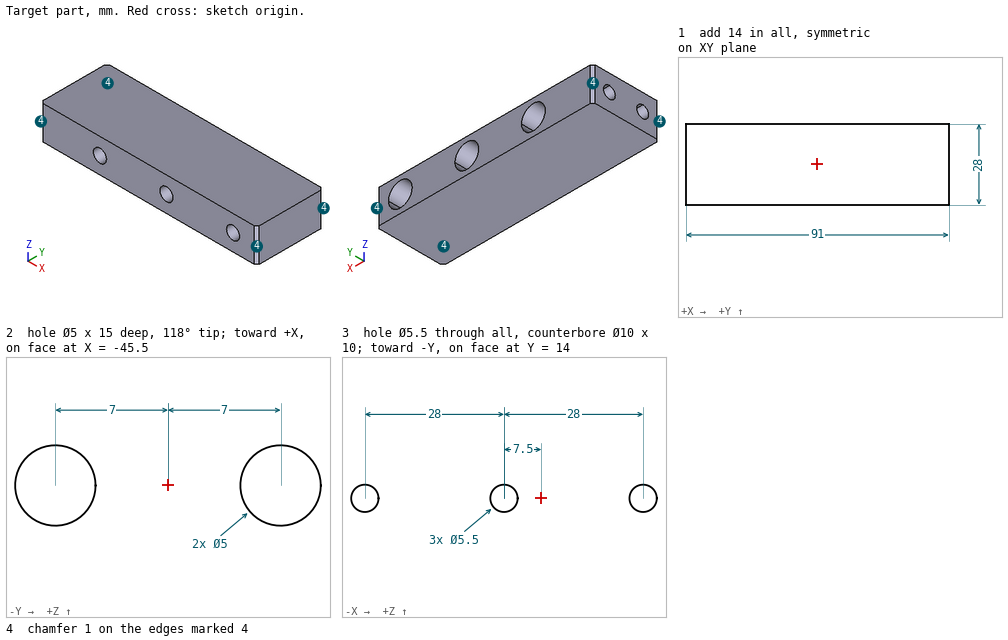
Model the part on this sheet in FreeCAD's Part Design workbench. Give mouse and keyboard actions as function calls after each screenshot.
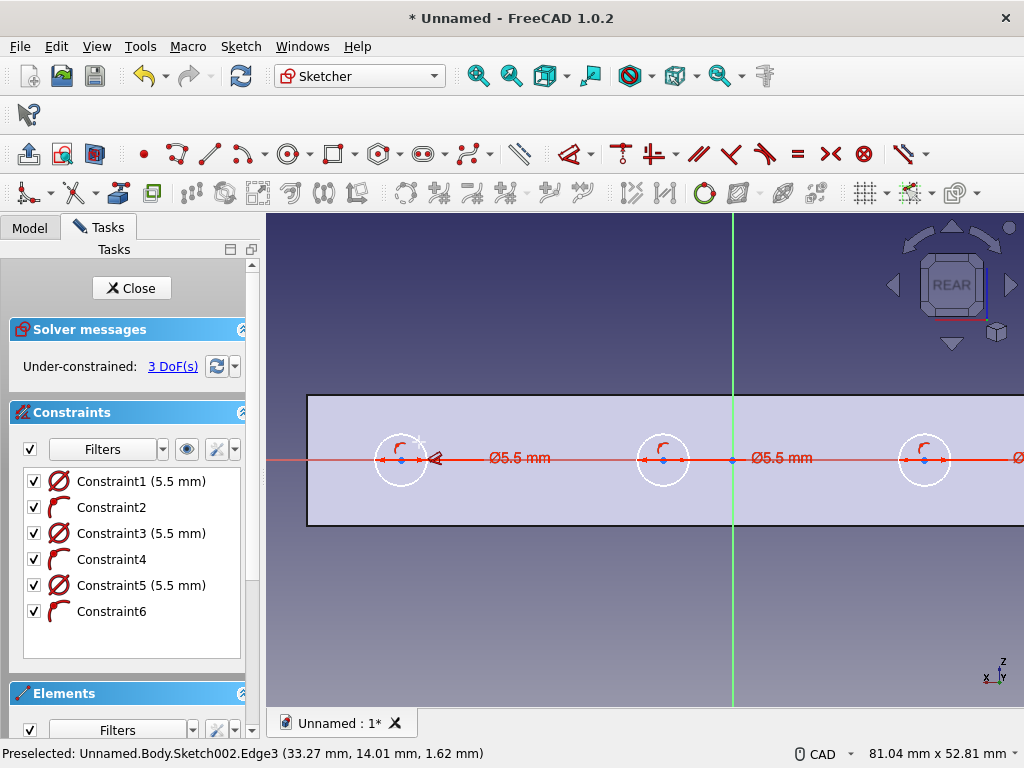
click(663, 460)
click(698, 494)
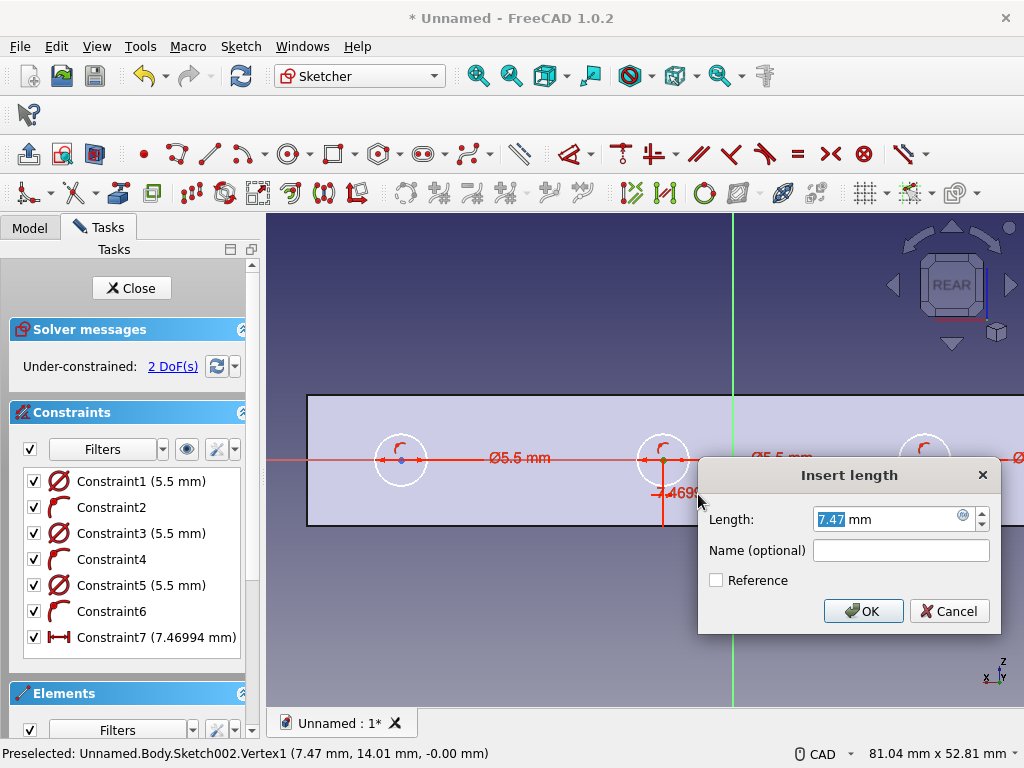
text(7.5)
key(Return)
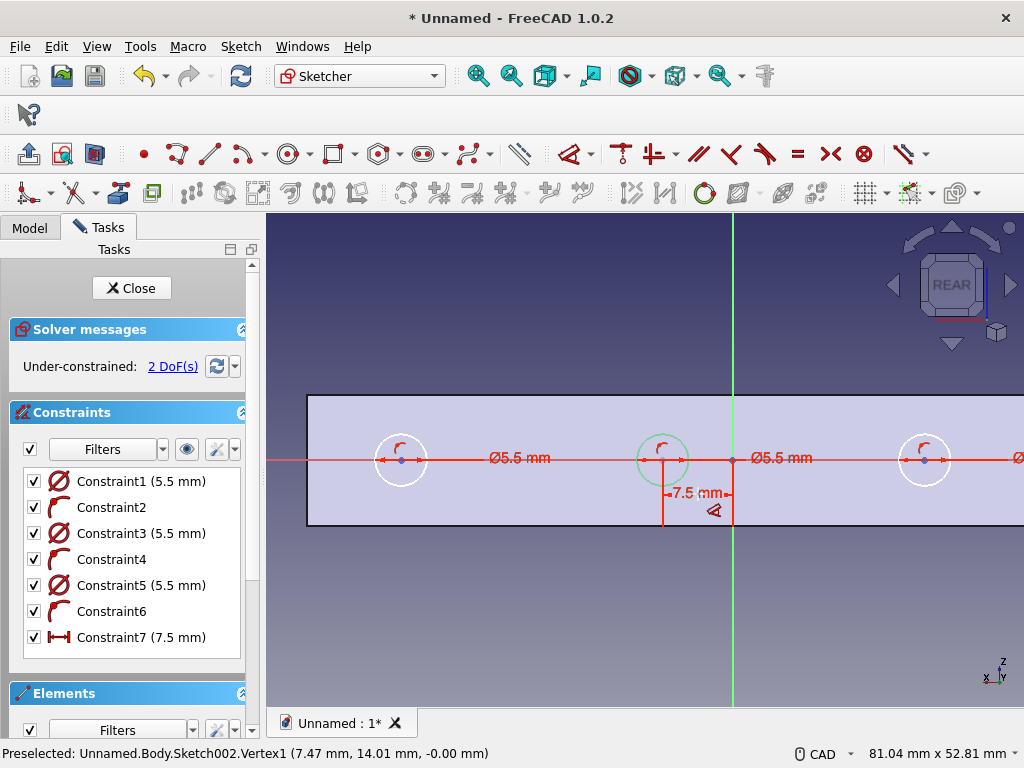
click(663, 460)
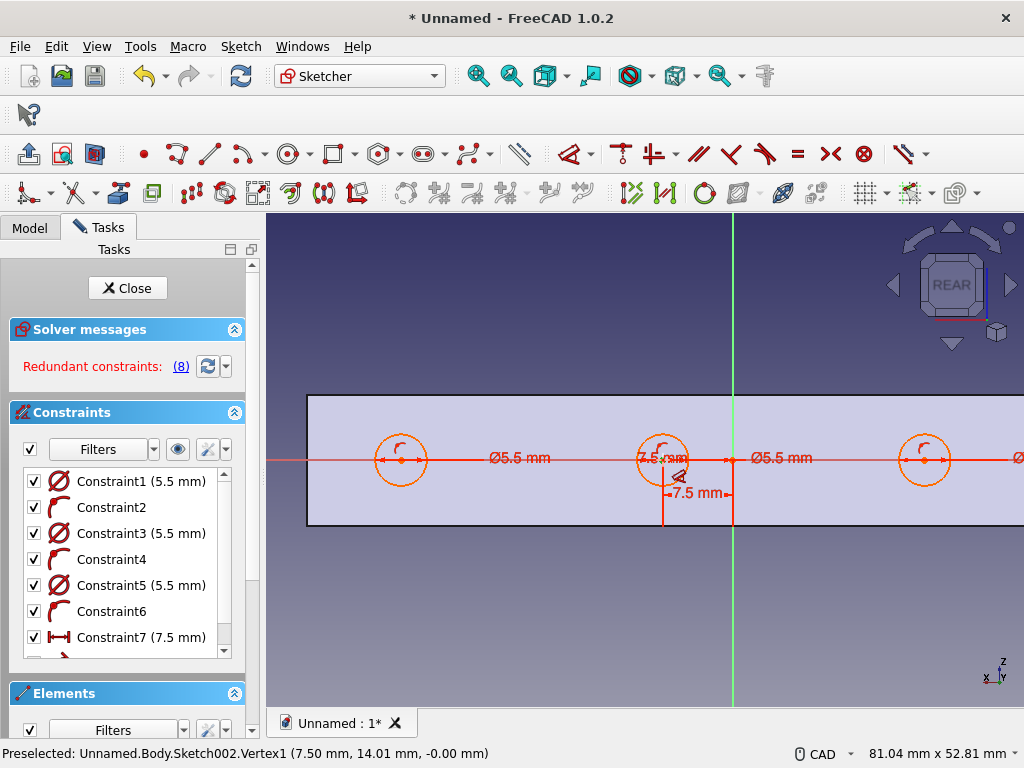
scroll(401, 460, down, 2)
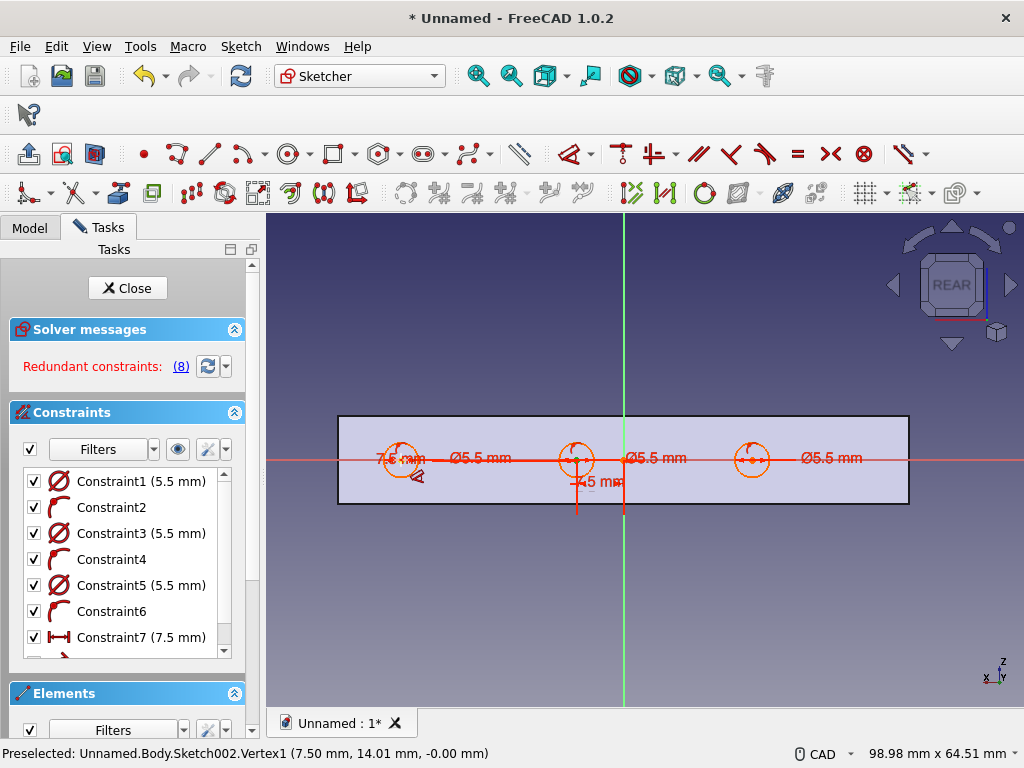
click(752, 460)
click(705, 494)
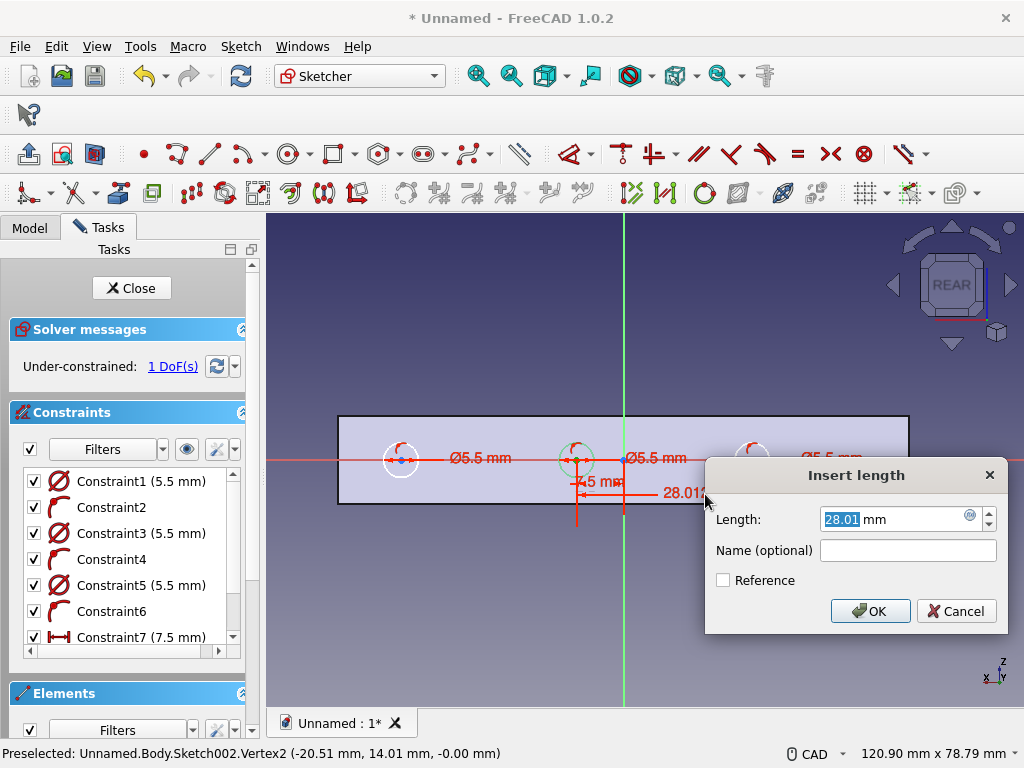
text(28)
key(Return)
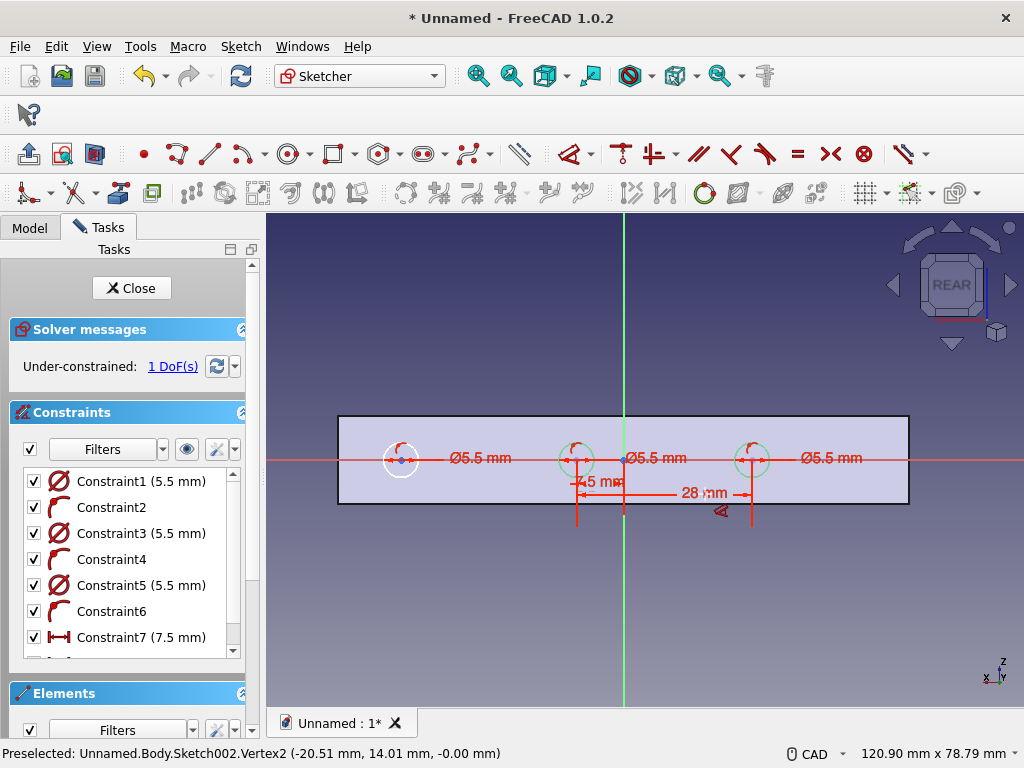
click(577, 460)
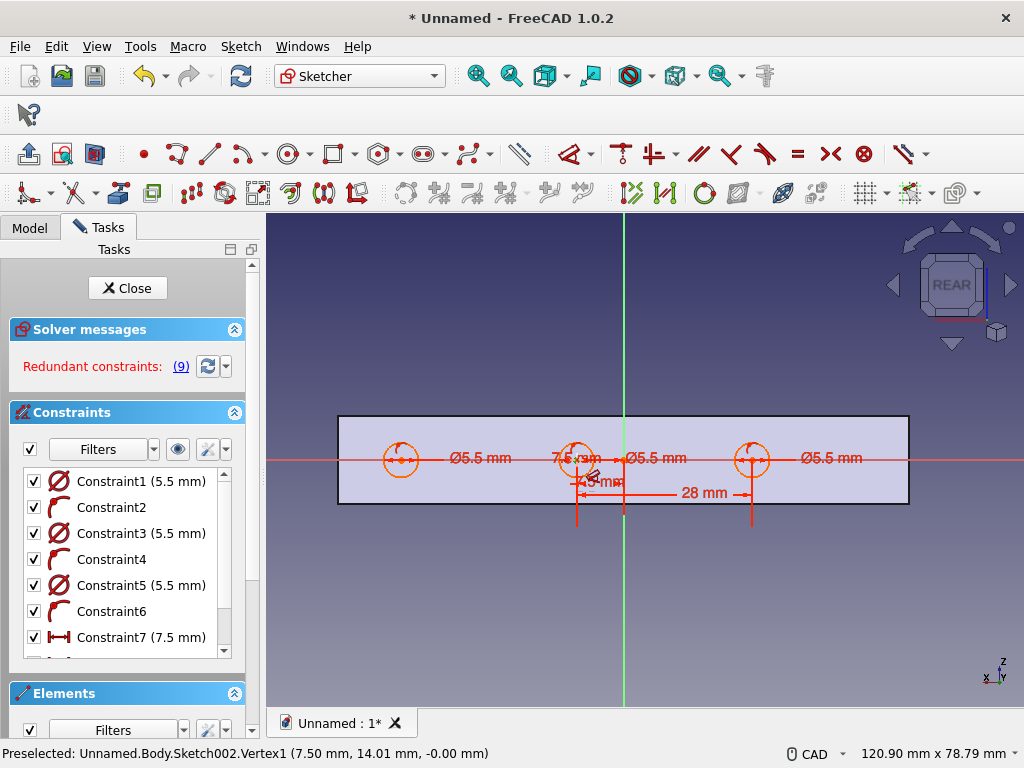
click(401, 460)
click(489, 494)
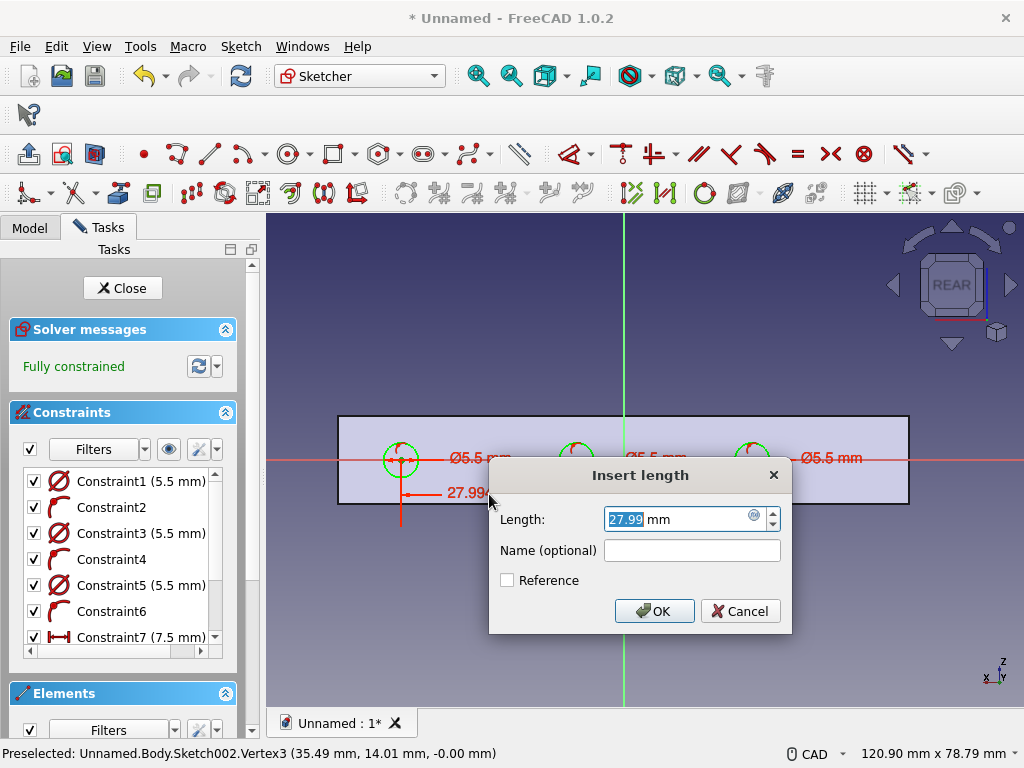
text(28)
key(Return)
key(Escape)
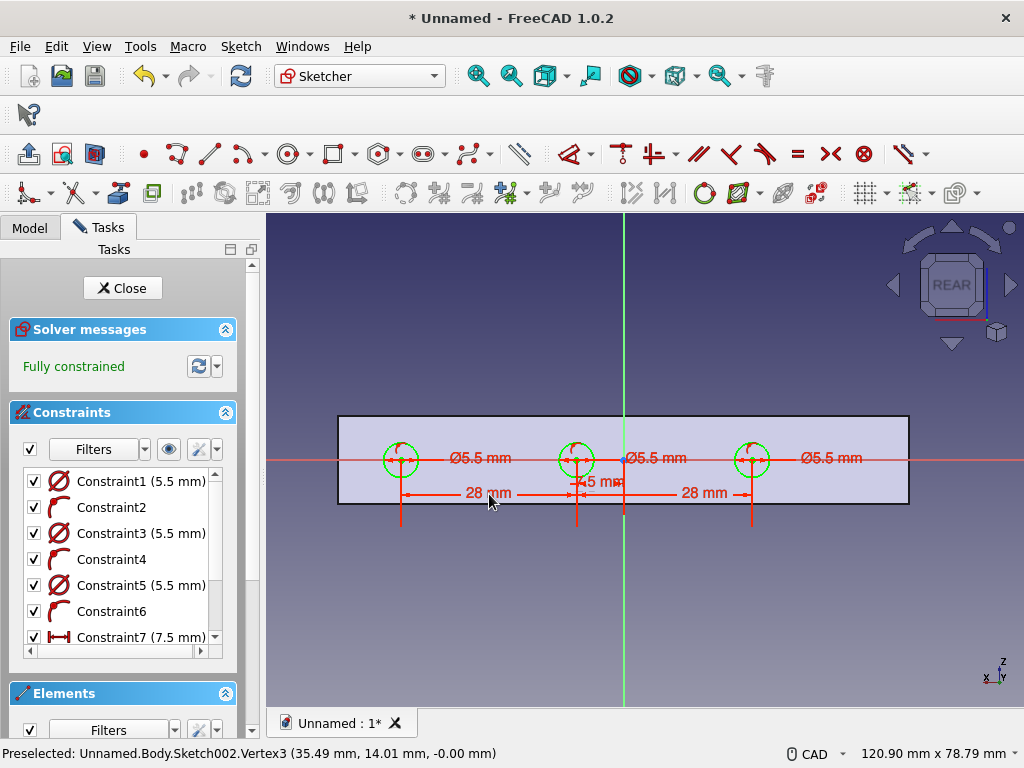
click(123, 288)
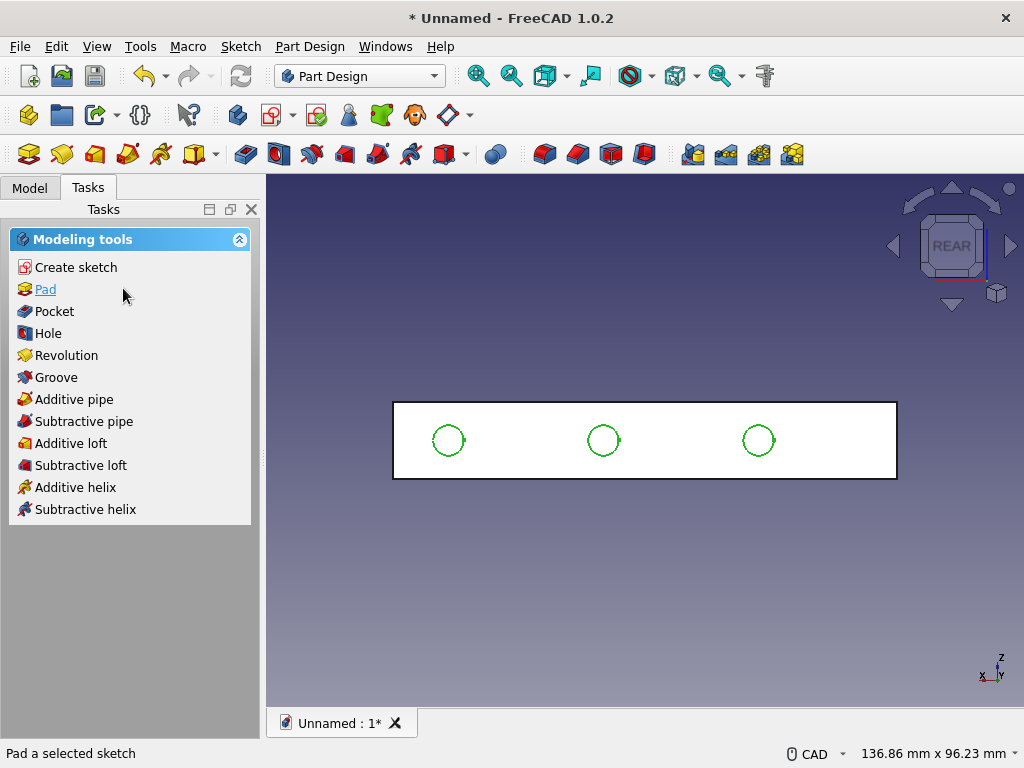
click(279, 154)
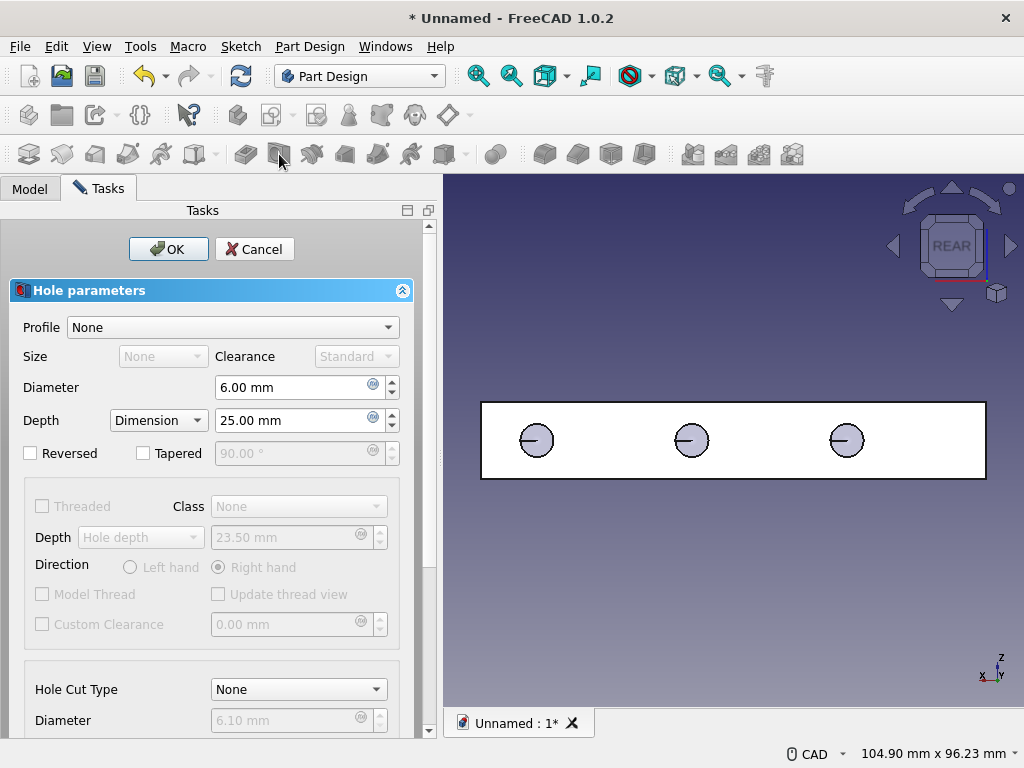
triple_click(300, 388)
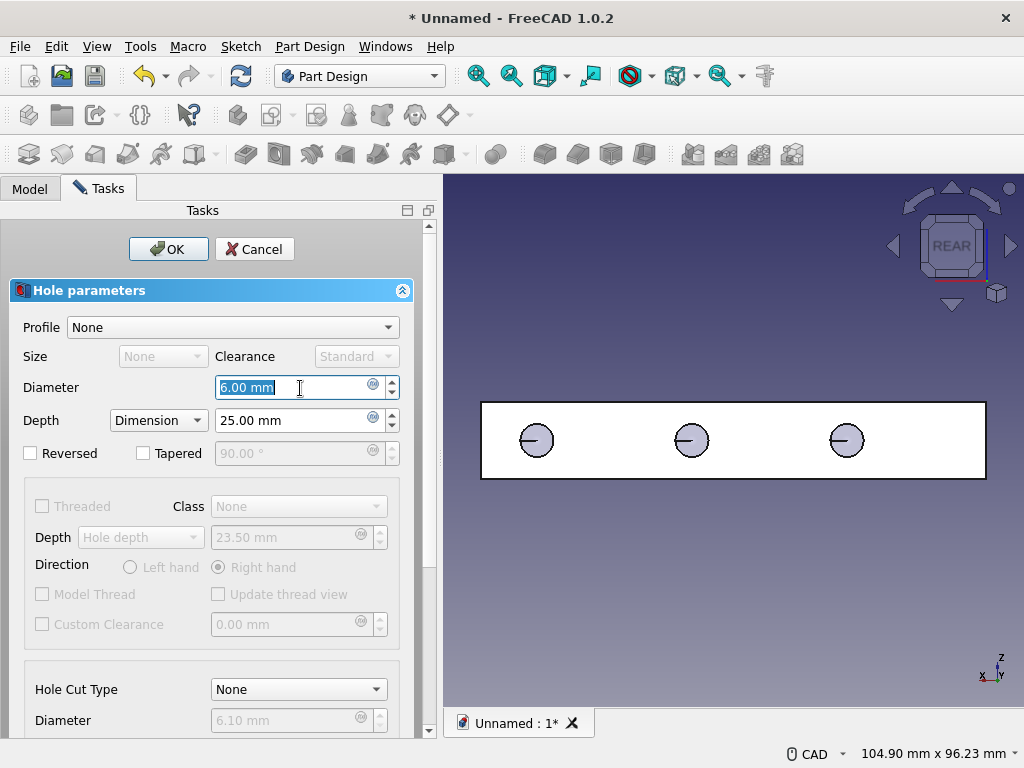
text(5.5)
key(Tab)